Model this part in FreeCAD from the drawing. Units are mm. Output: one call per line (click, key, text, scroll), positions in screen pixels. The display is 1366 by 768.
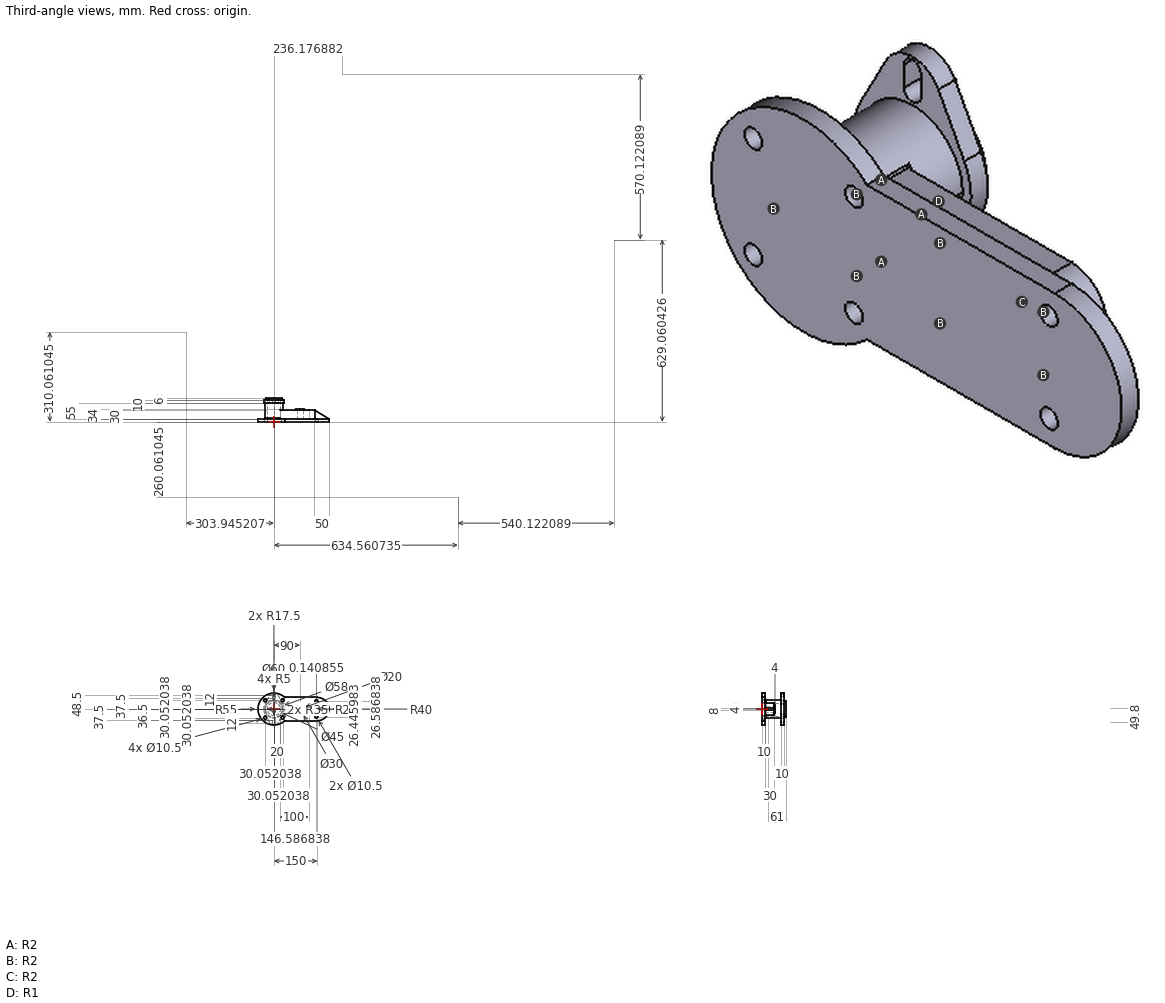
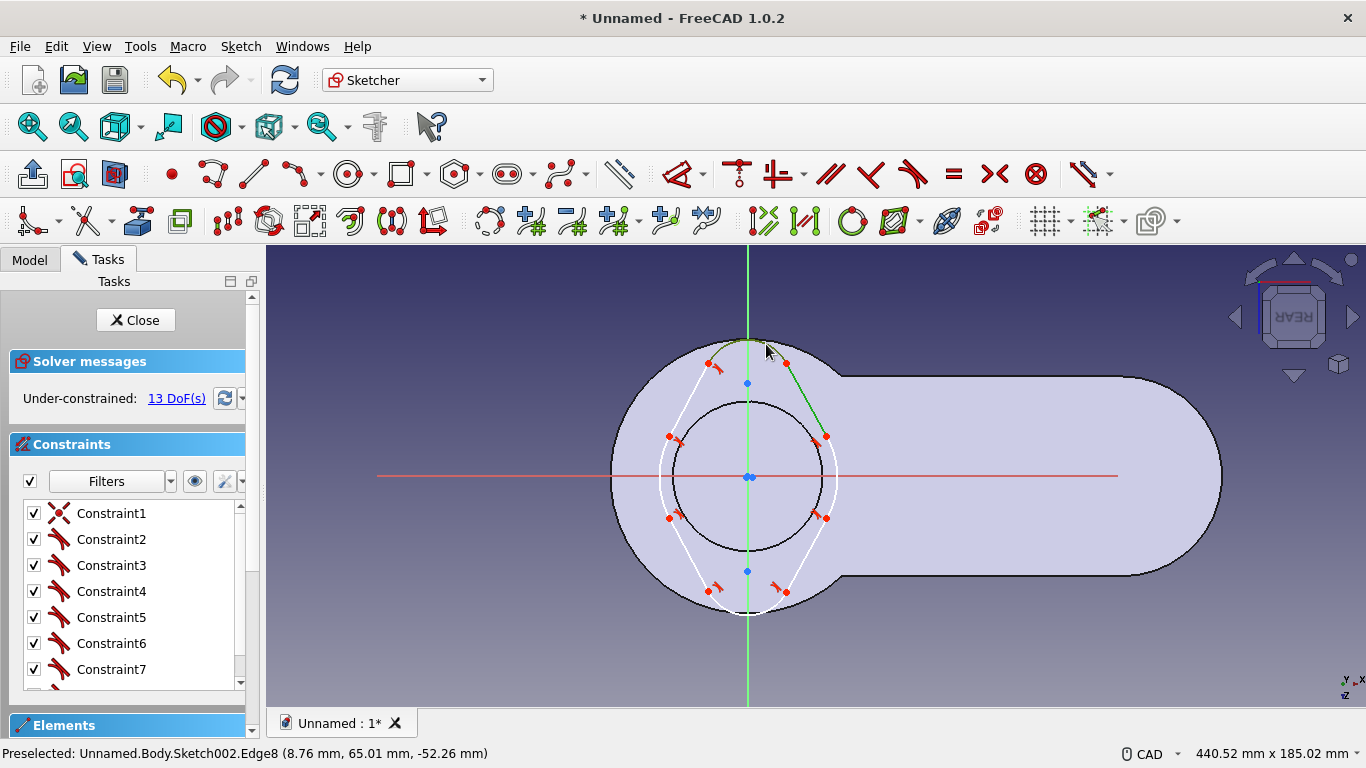
key(t)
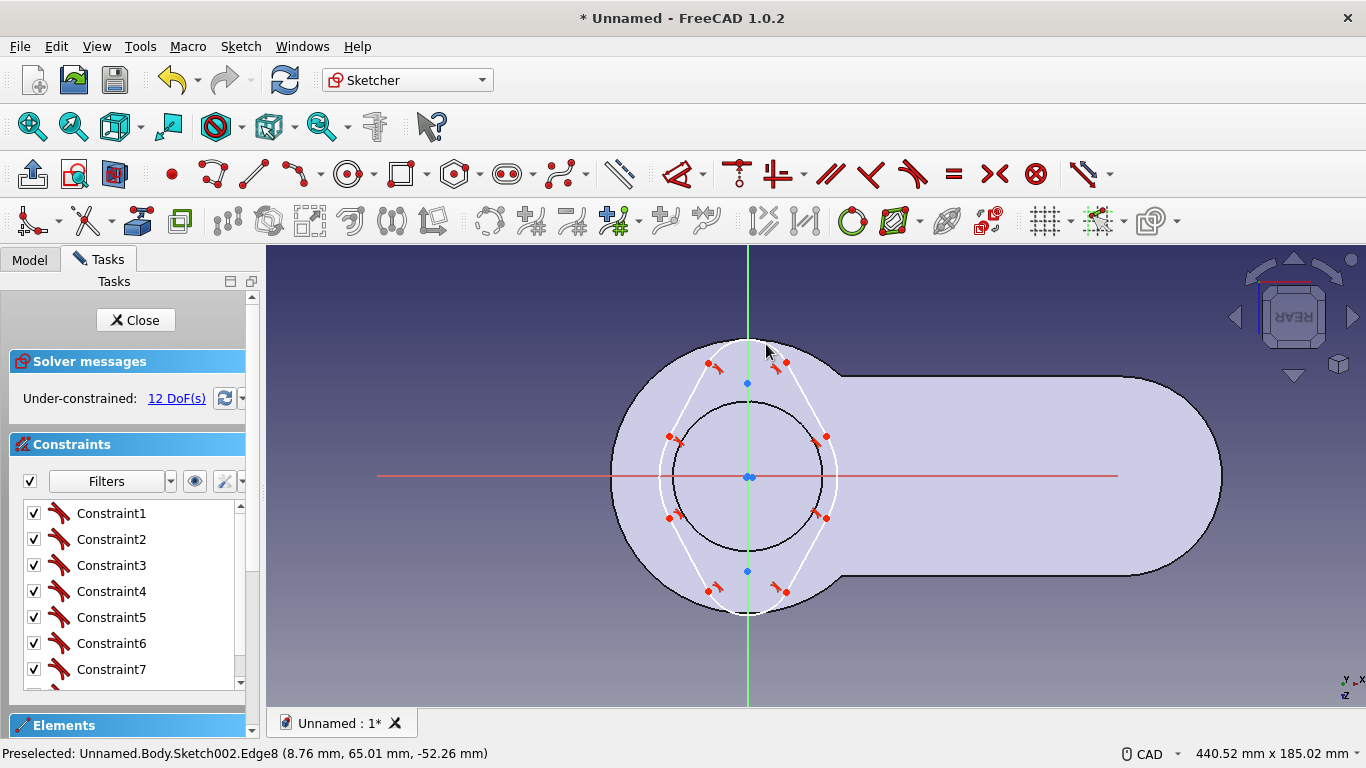
click(661, 461)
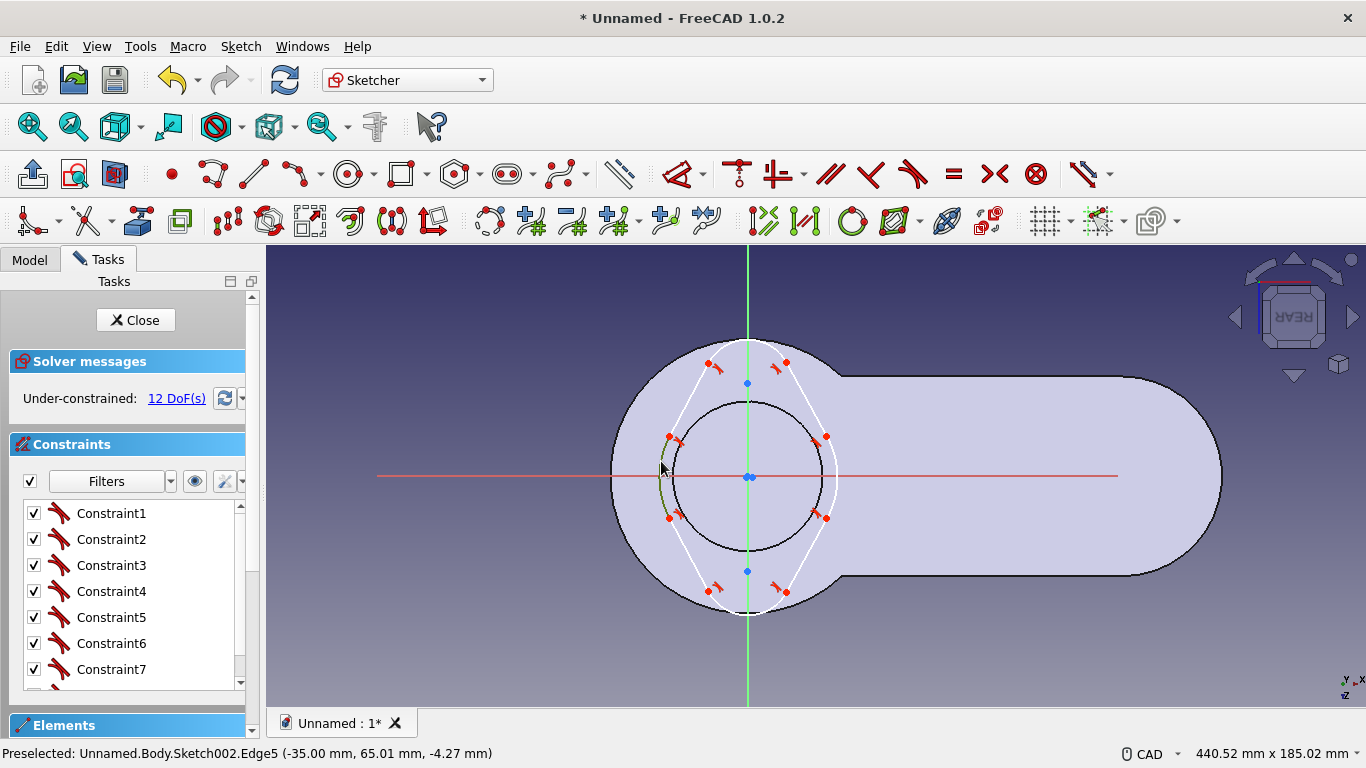
click(836, 495)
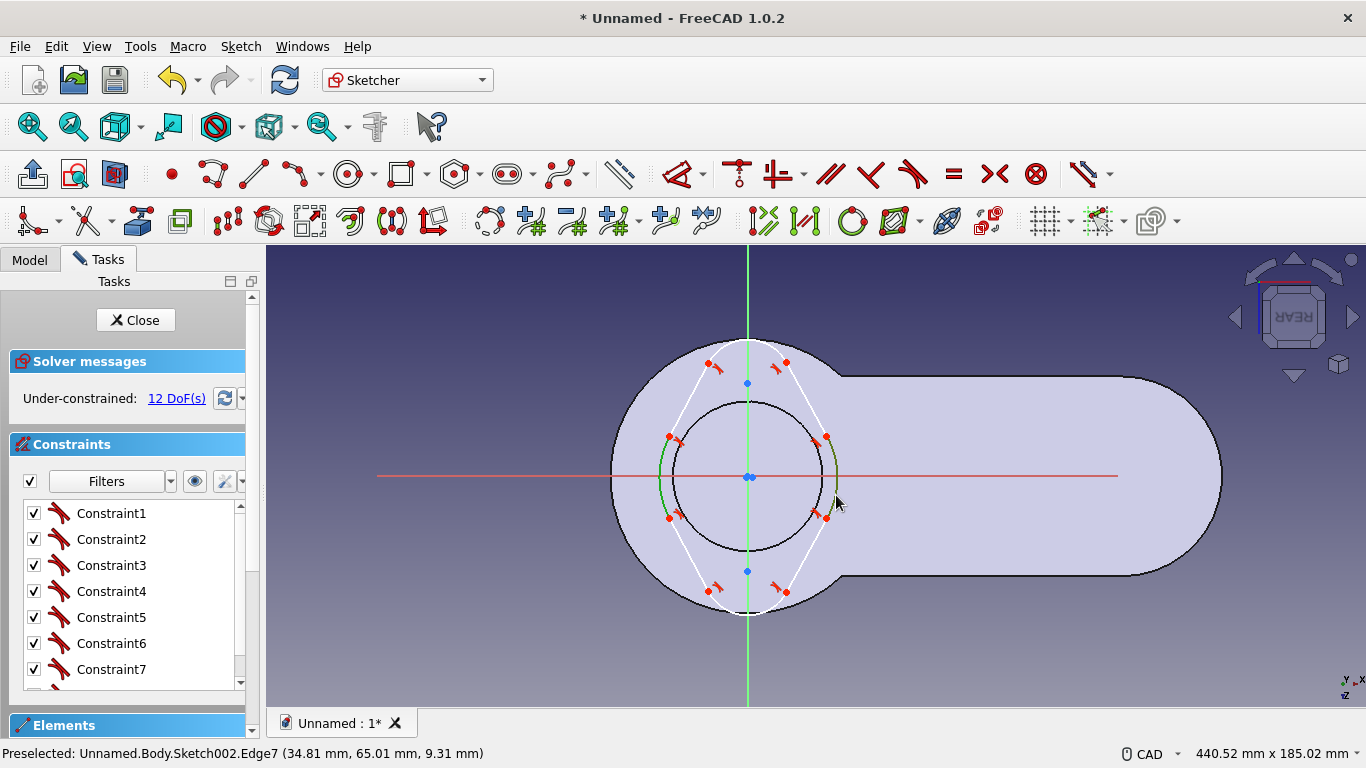
click(737, 174)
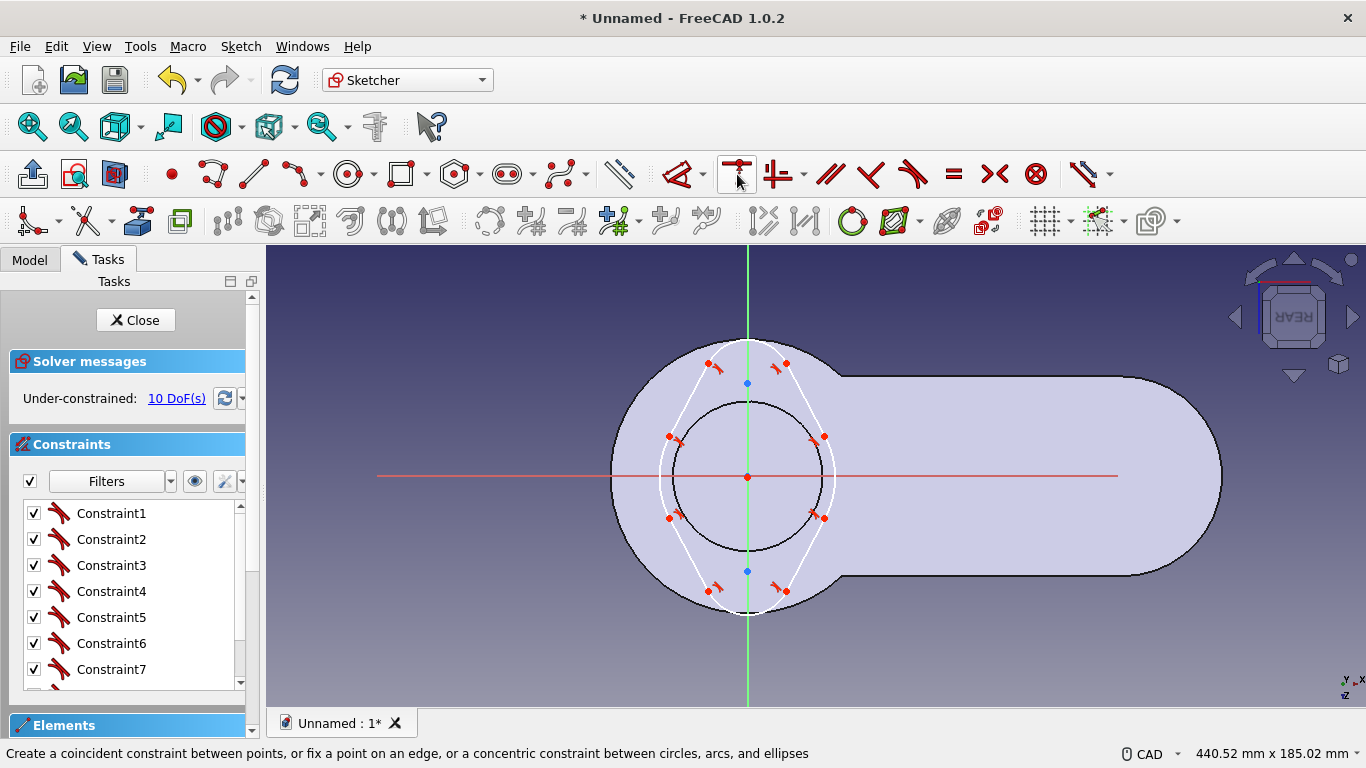
drag(737, 466, 758, 488)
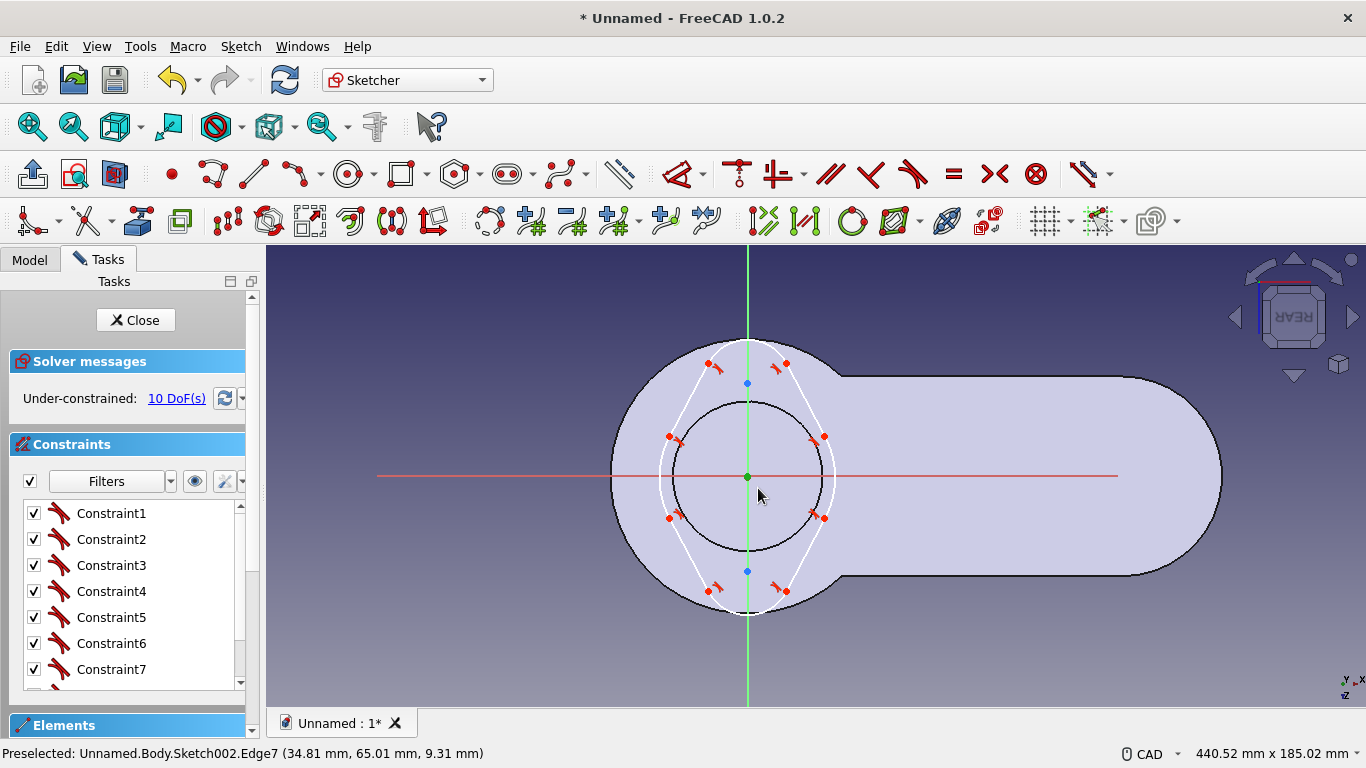
key(c)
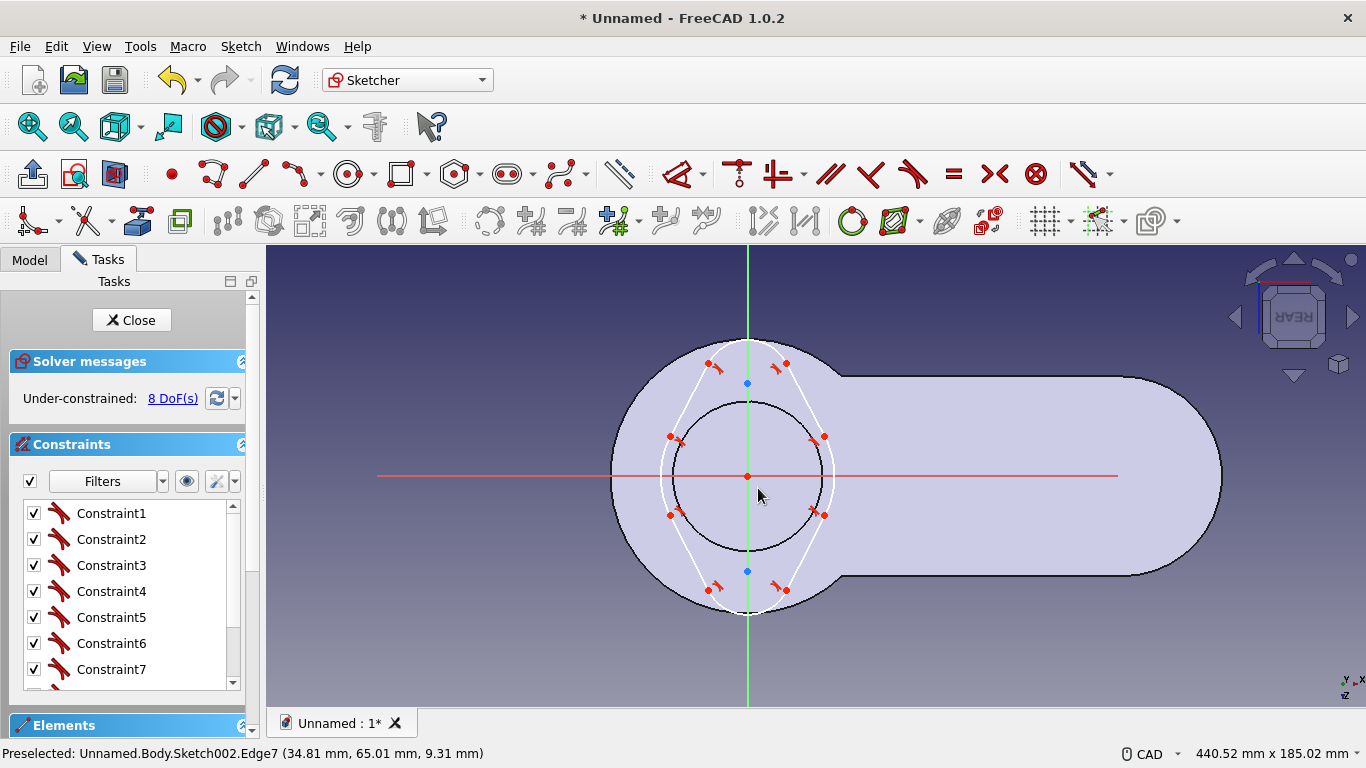
click(662, 459)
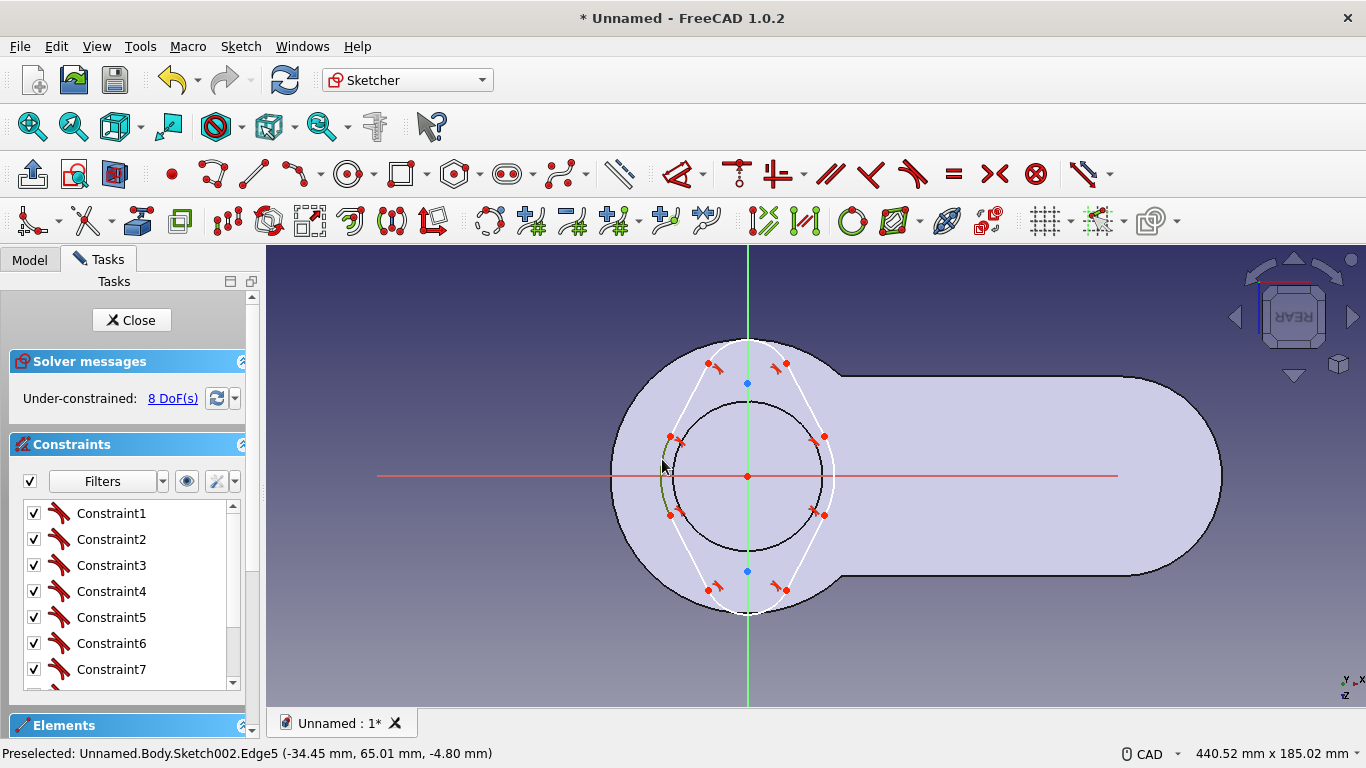
click(833, 492)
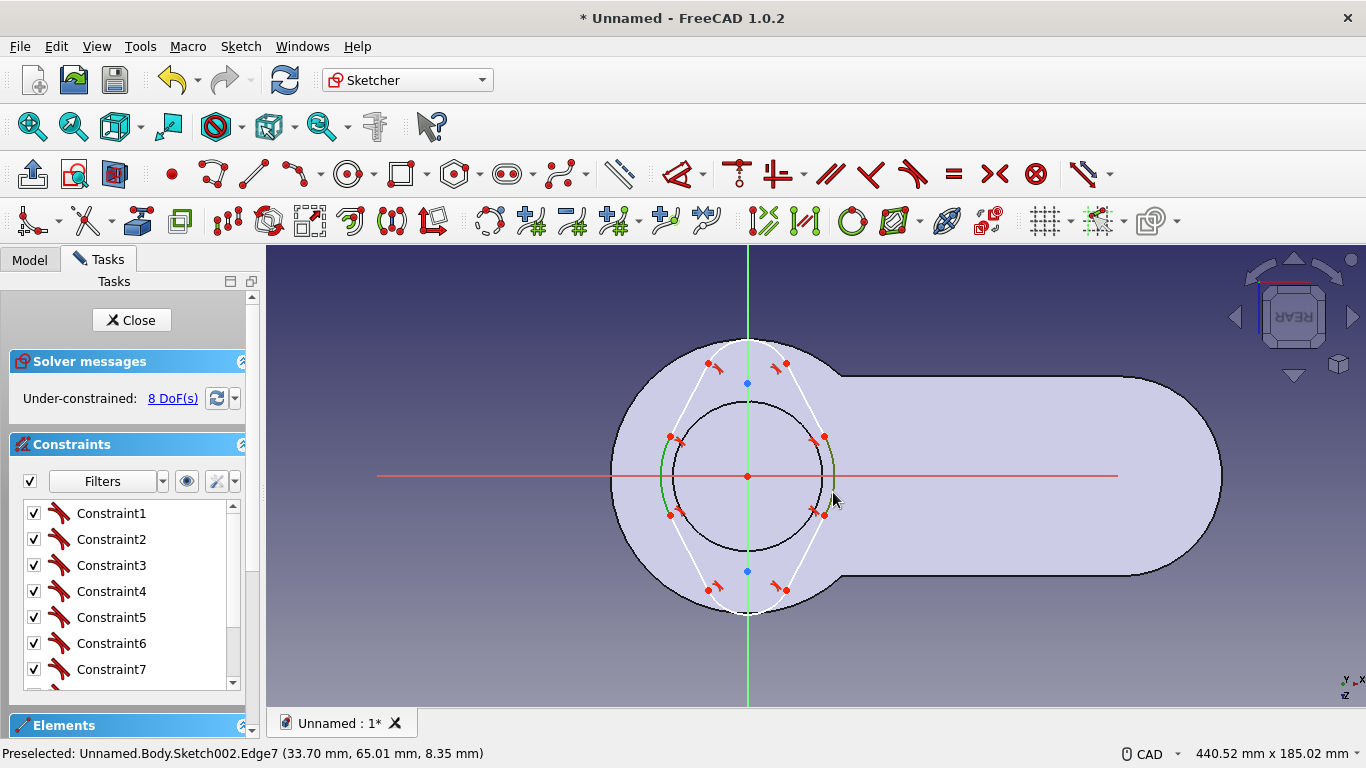
key(e)